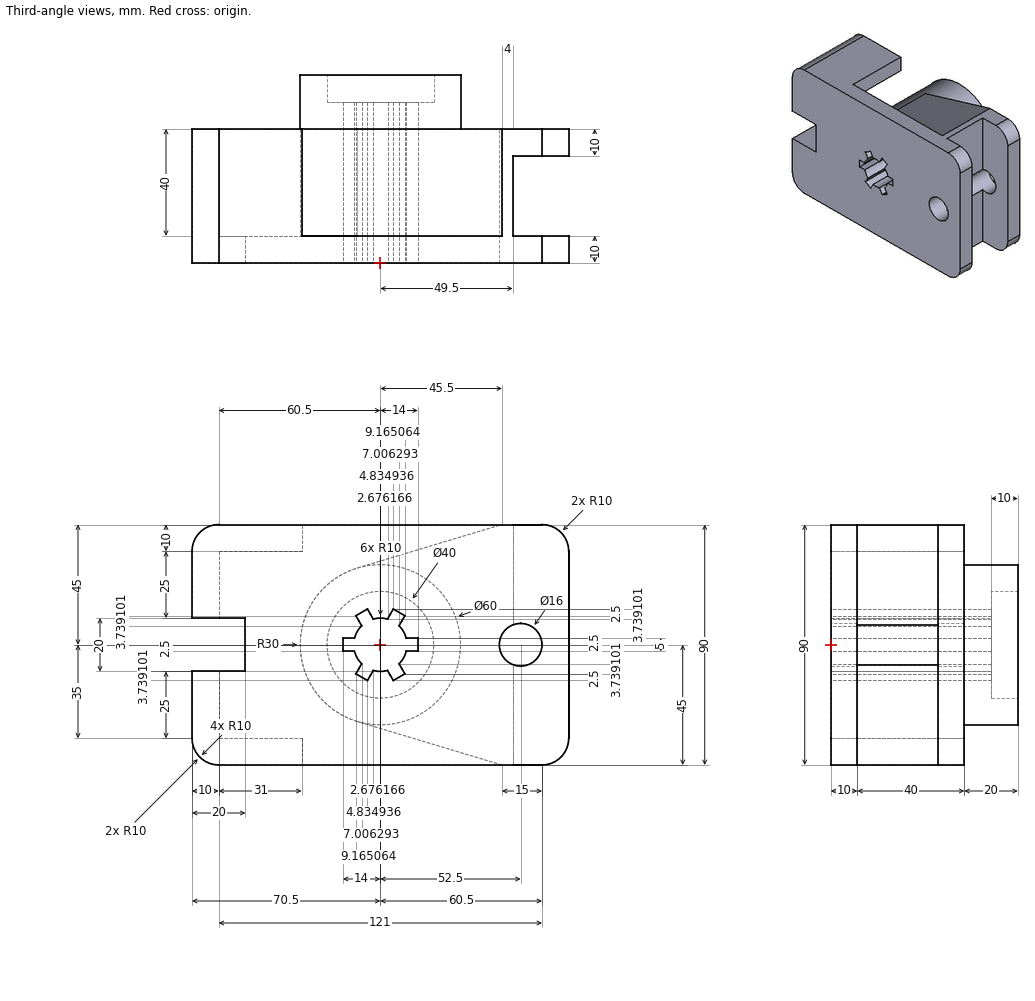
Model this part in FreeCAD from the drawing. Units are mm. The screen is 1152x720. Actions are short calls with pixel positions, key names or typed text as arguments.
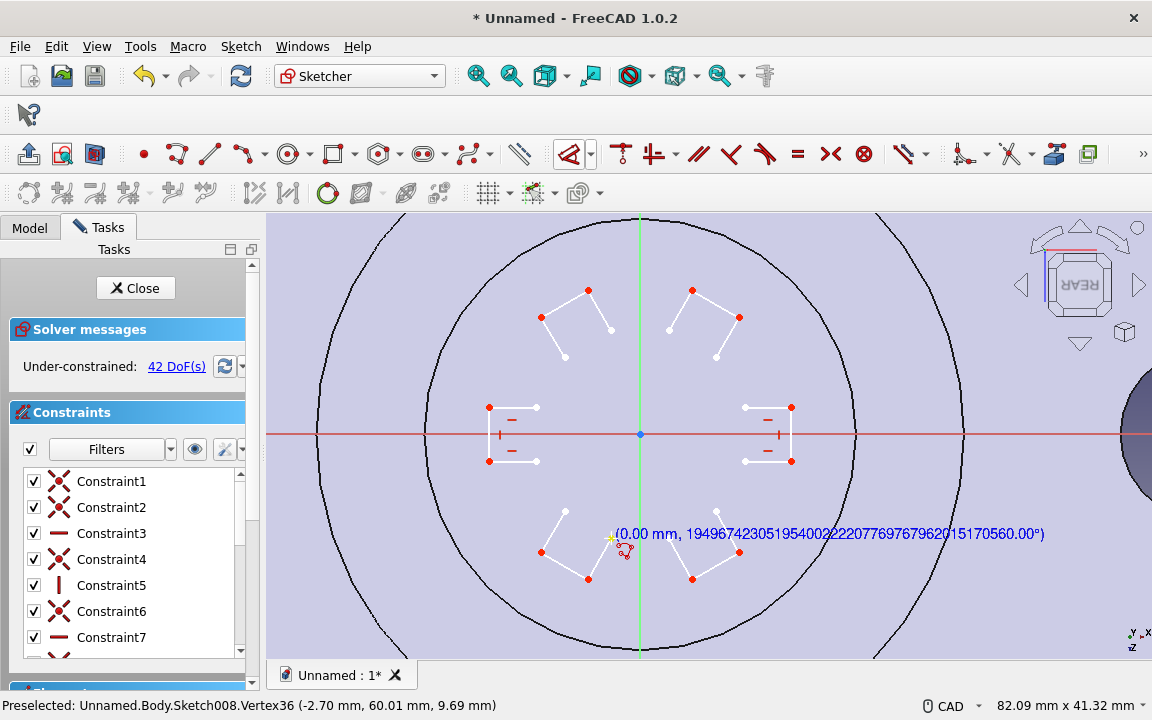
click(242, 154)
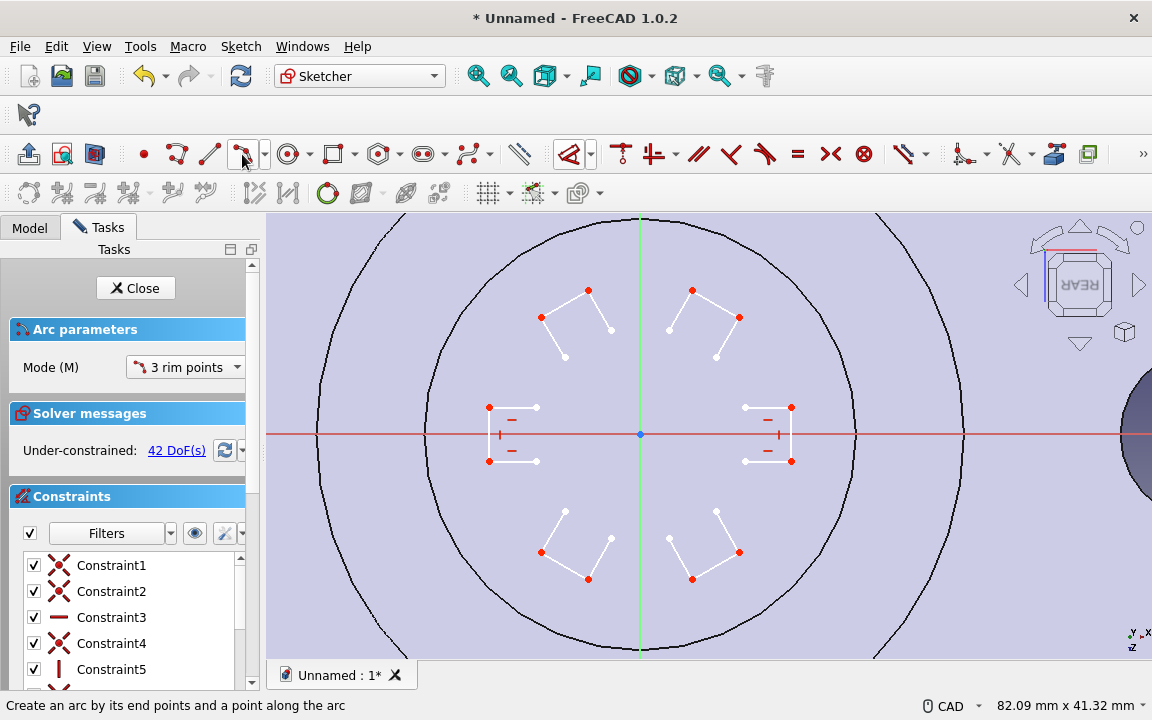
click(716, 512)
click(745, 462)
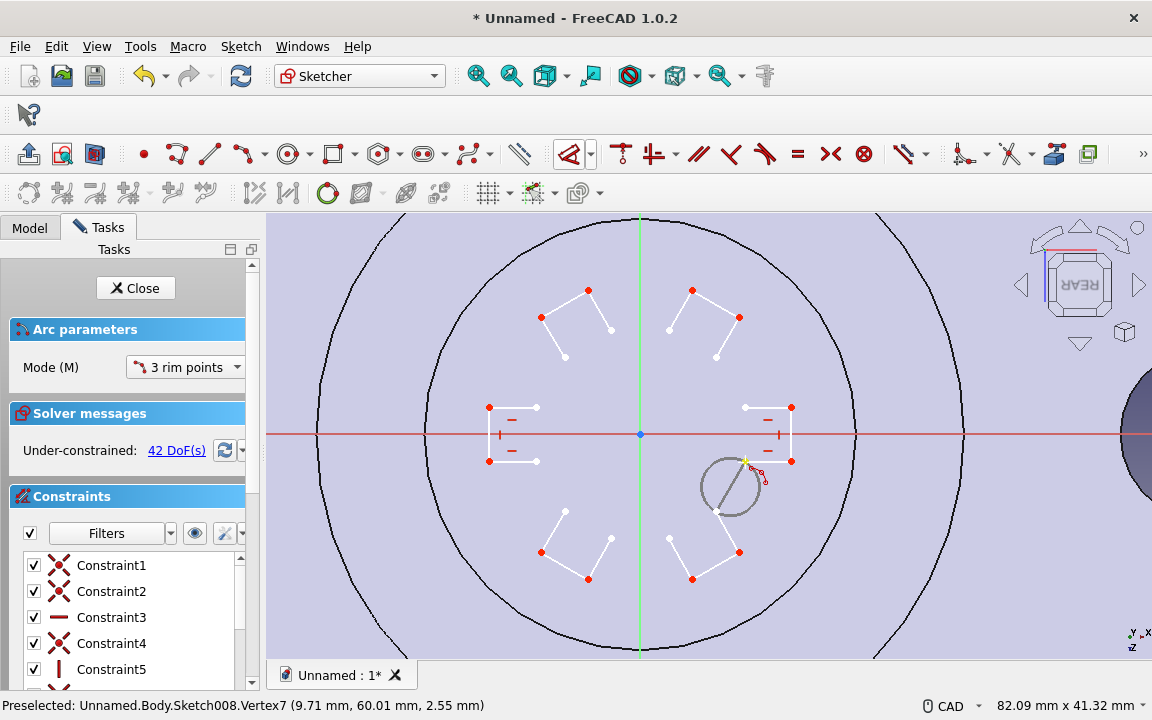
scroll(734, 488, up, 7)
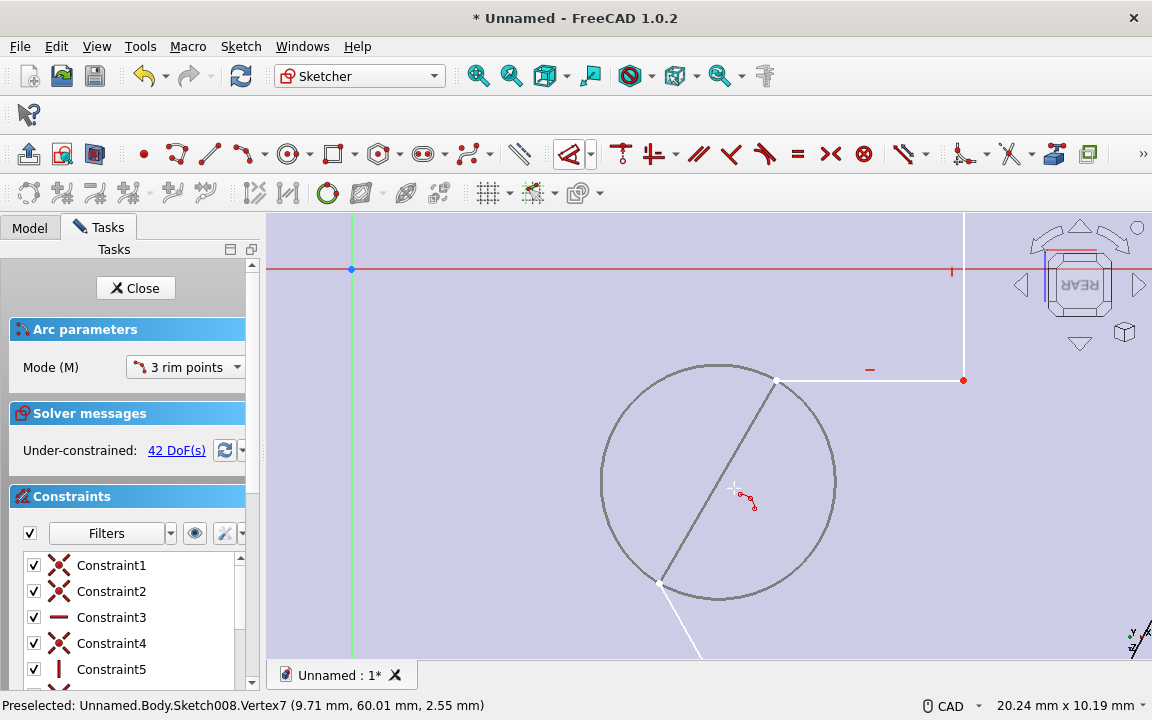
click(731, 488)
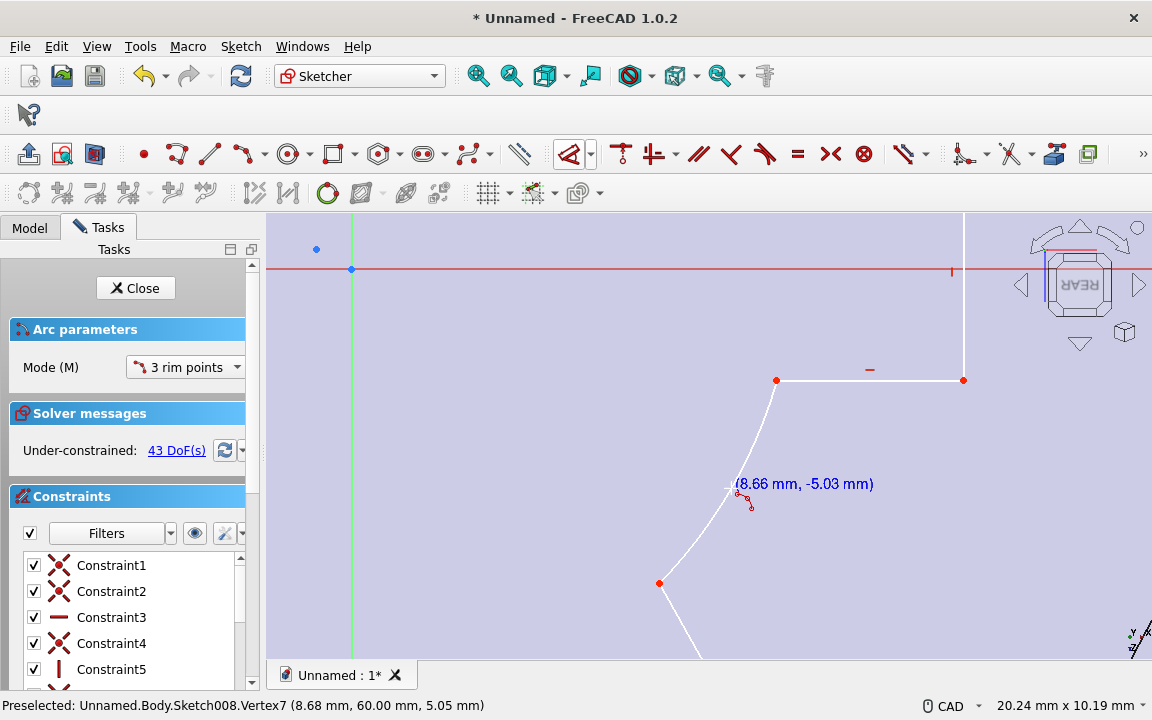
scroll(735, 491, down, 7)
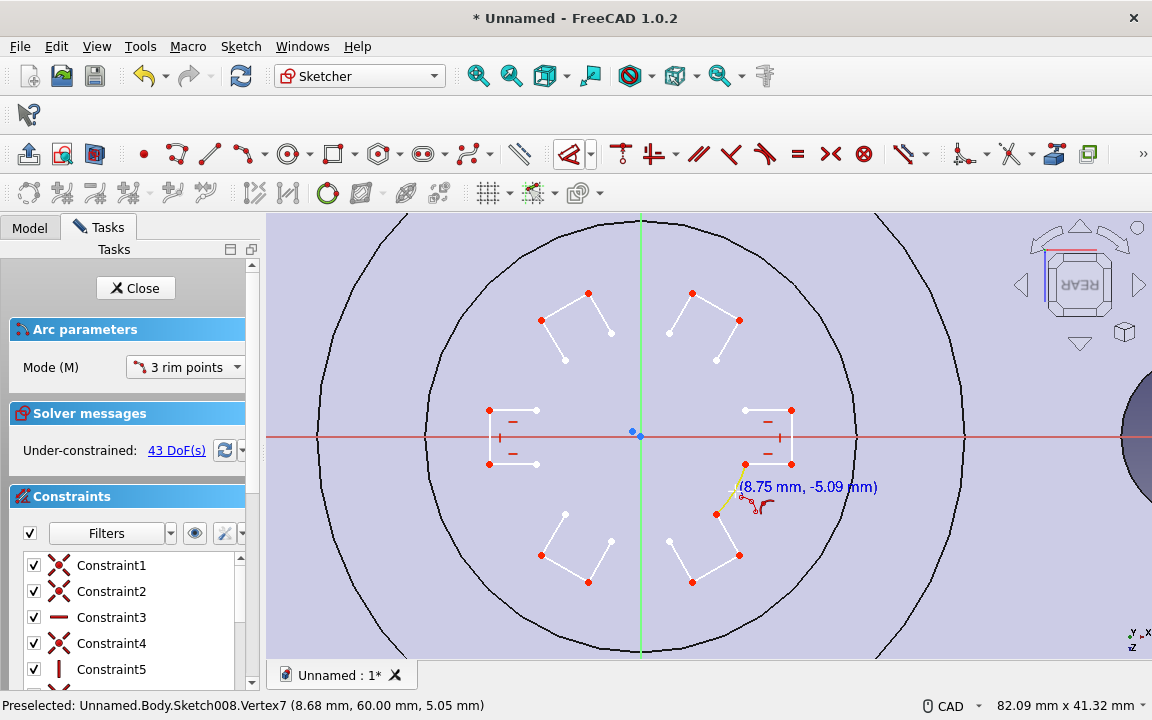
click(746, 410)
click(717, 360)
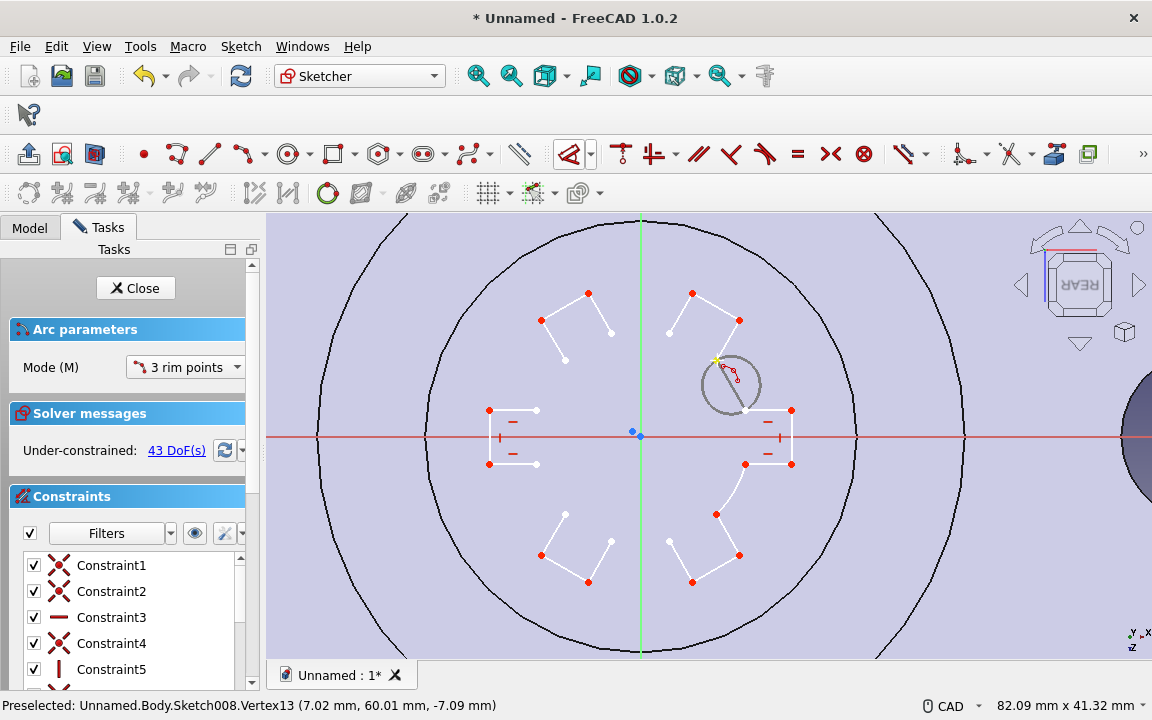
scroll(734, 383, up, 7)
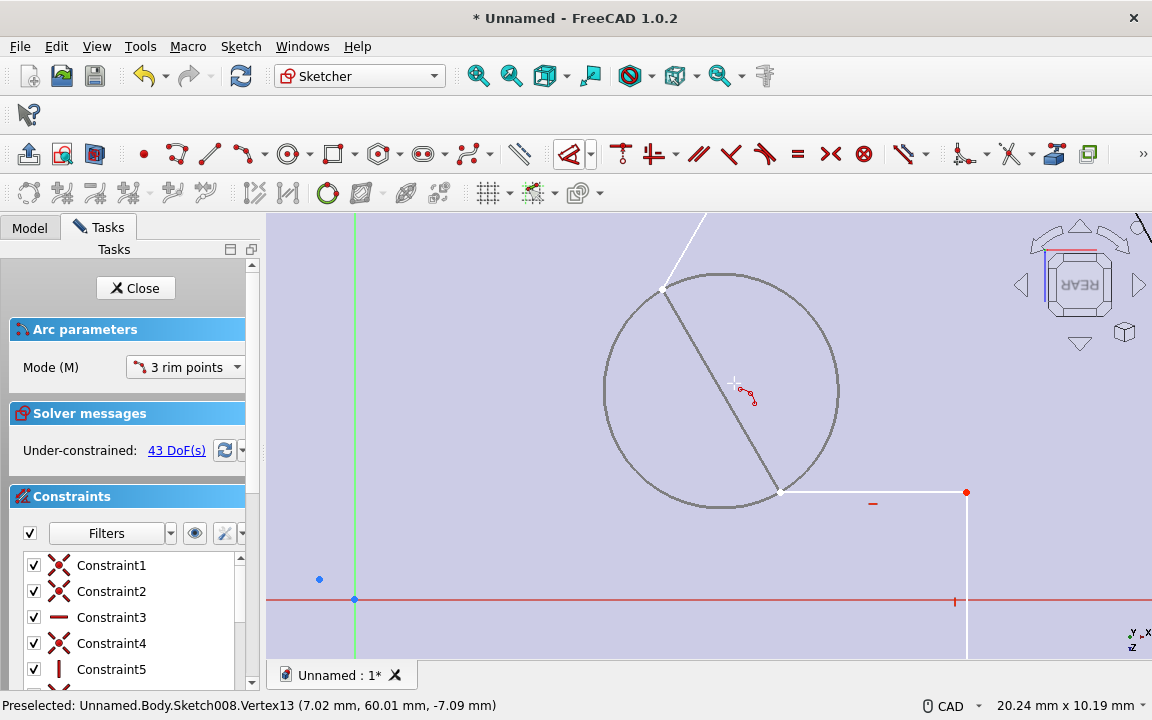
click(734, 381)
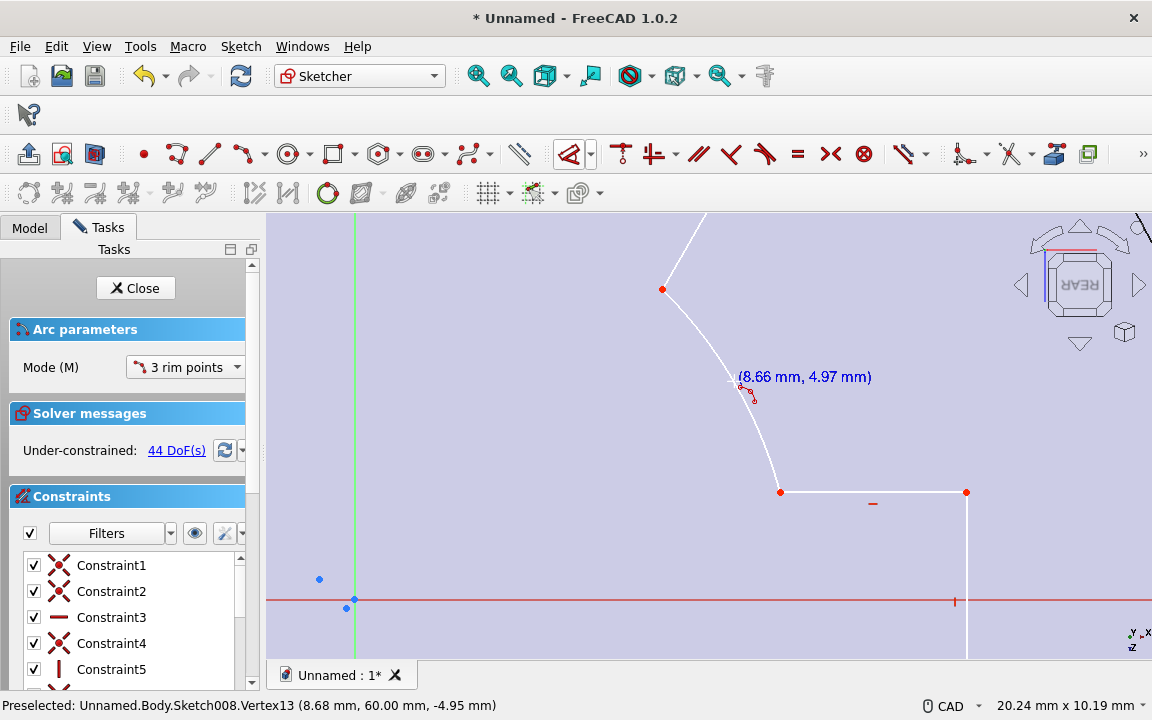
scroll(734, 382, down, 7)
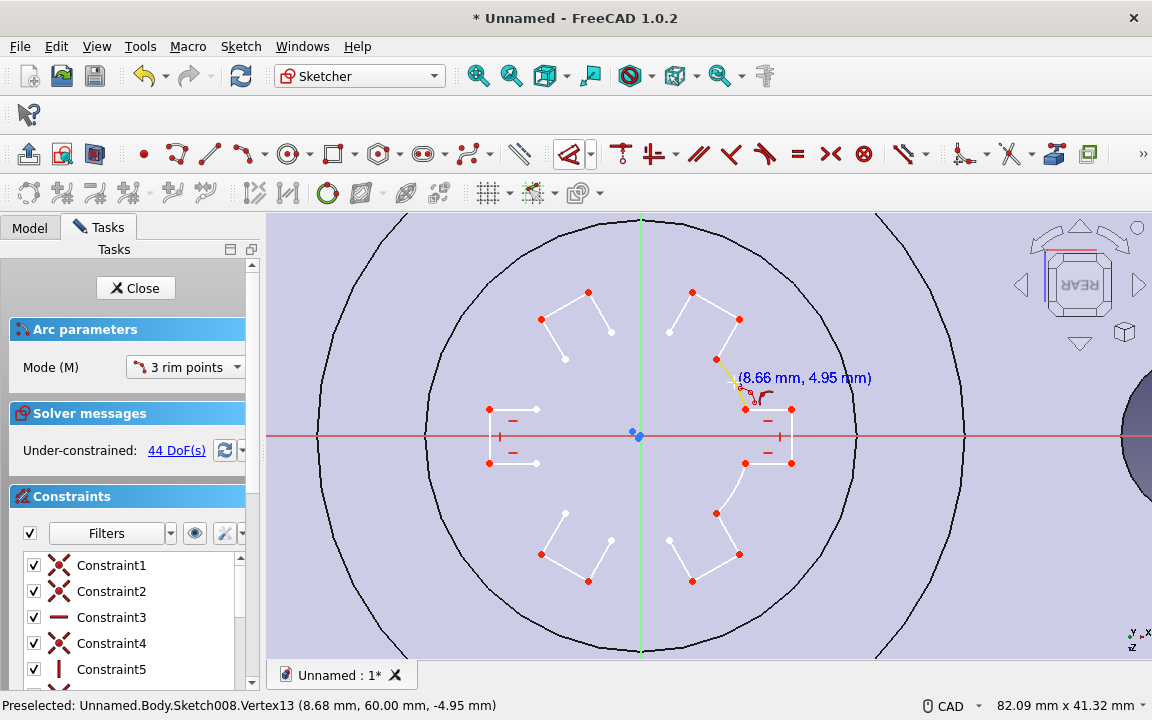
click(670, 333)
click(612, 333)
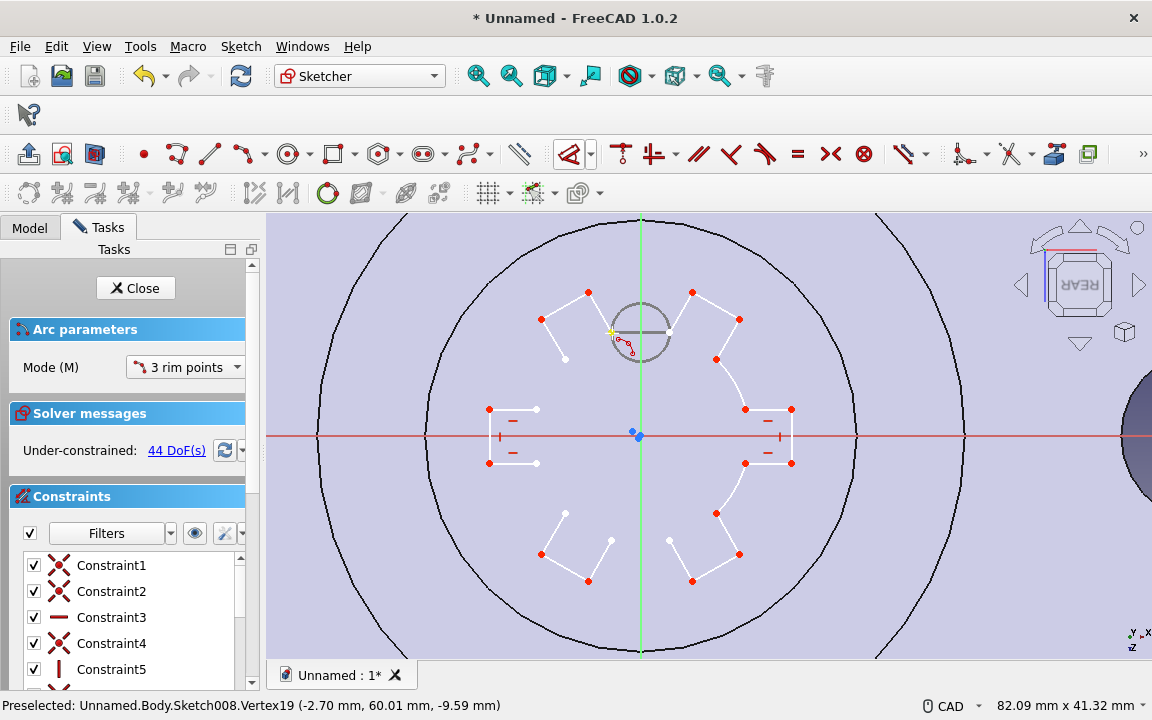
scroll(647, 328, up, 8)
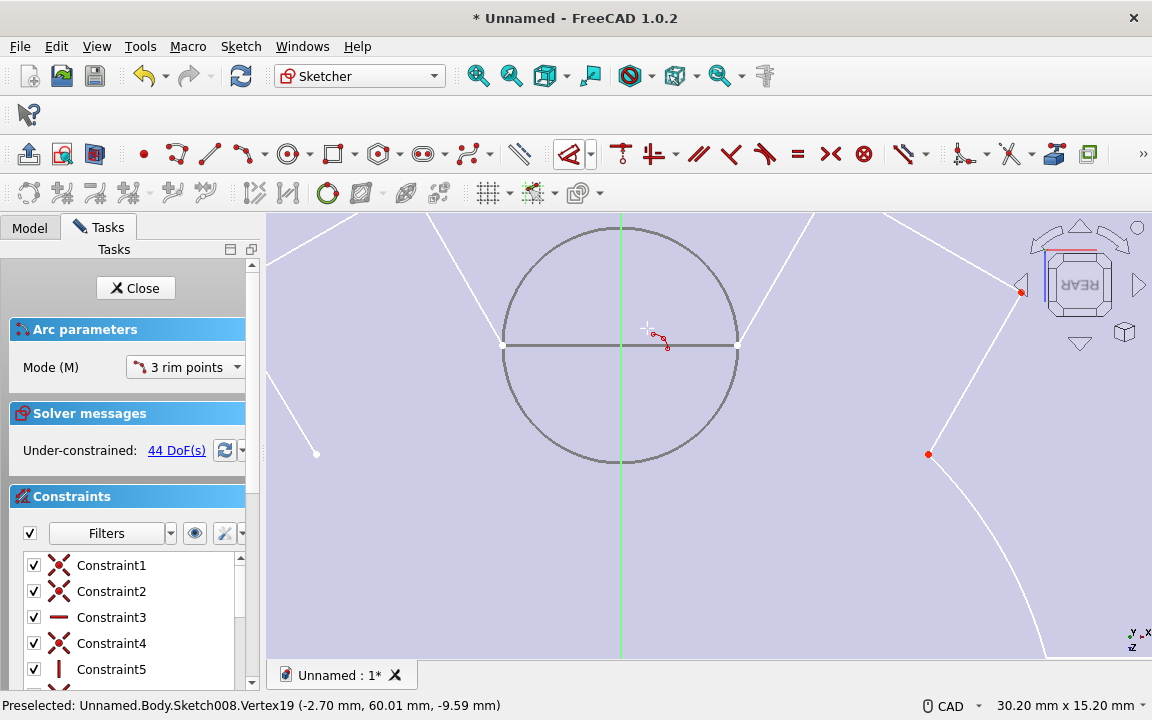
click(644, 328)